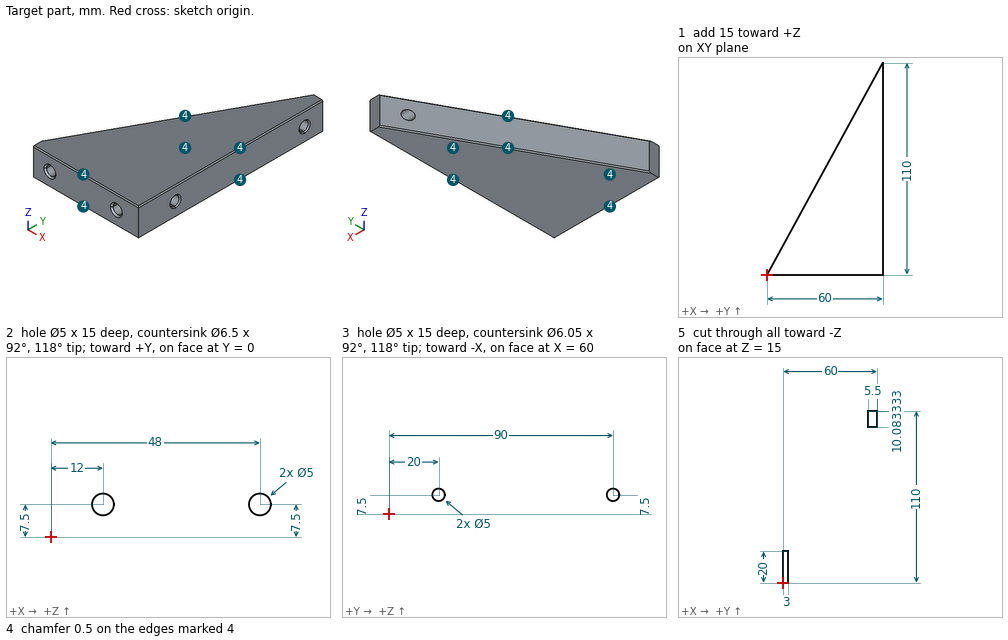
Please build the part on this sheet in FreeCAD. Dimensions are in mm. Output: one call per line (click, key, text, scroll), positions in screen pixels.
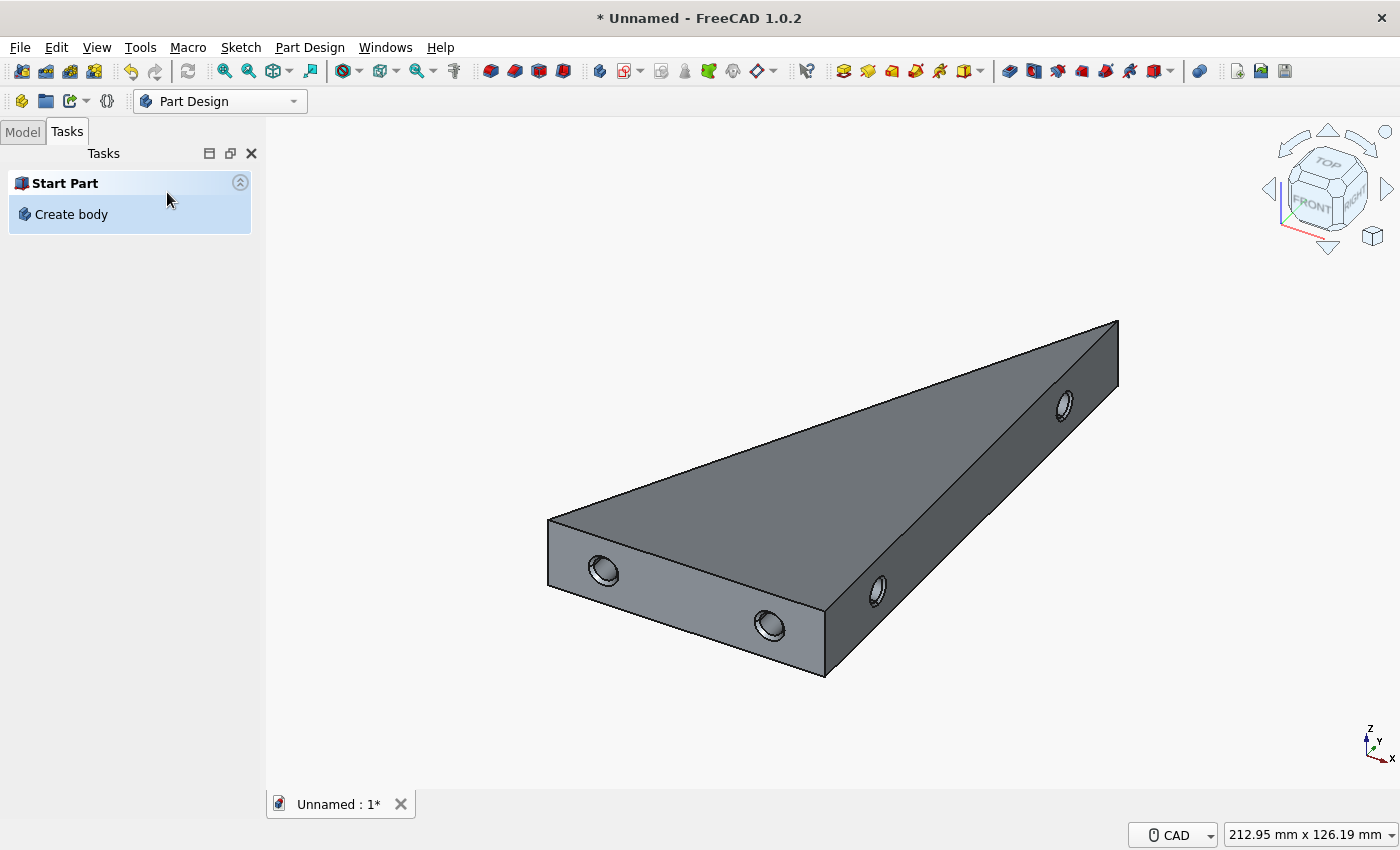
click(789, 516)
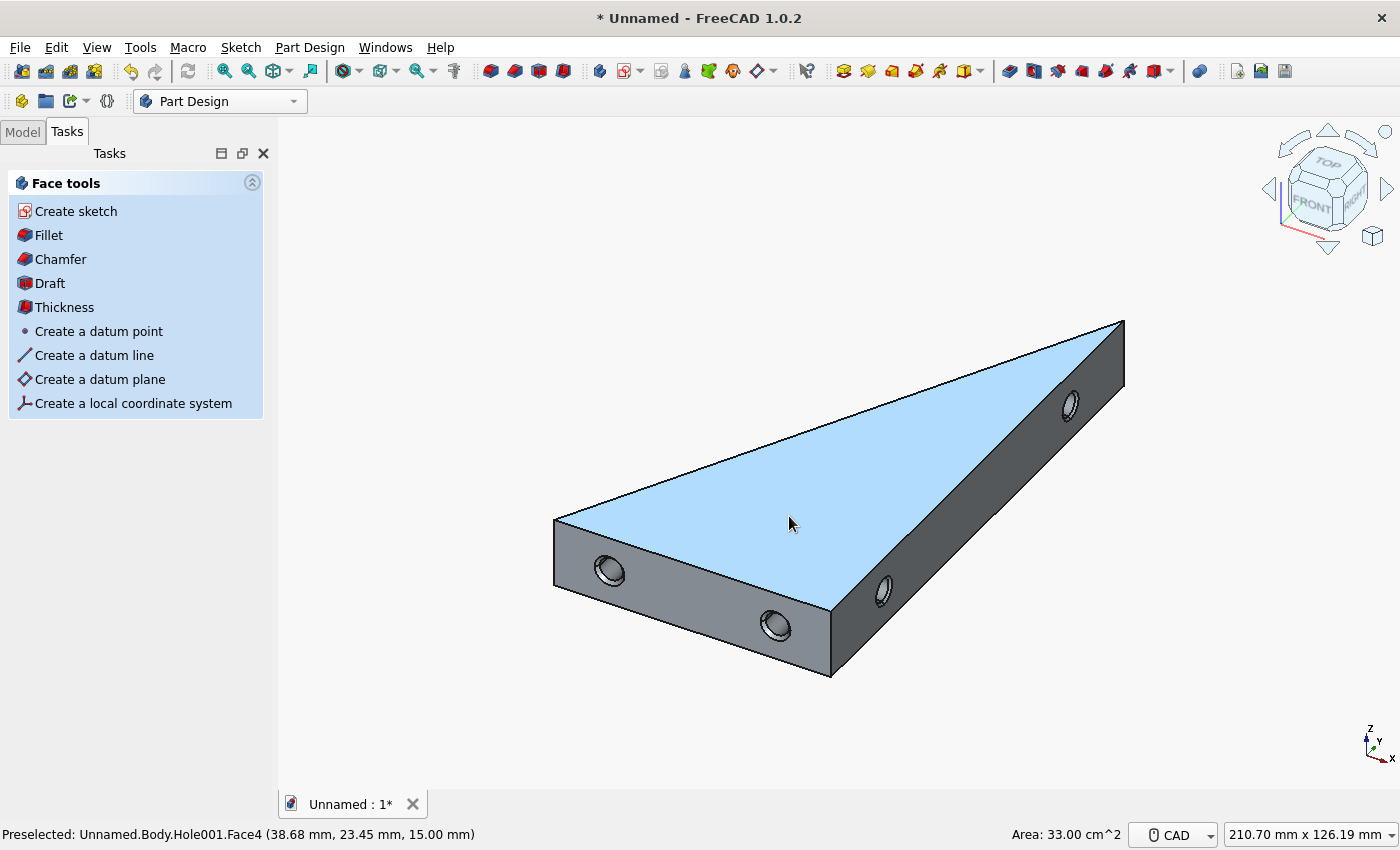
key(0)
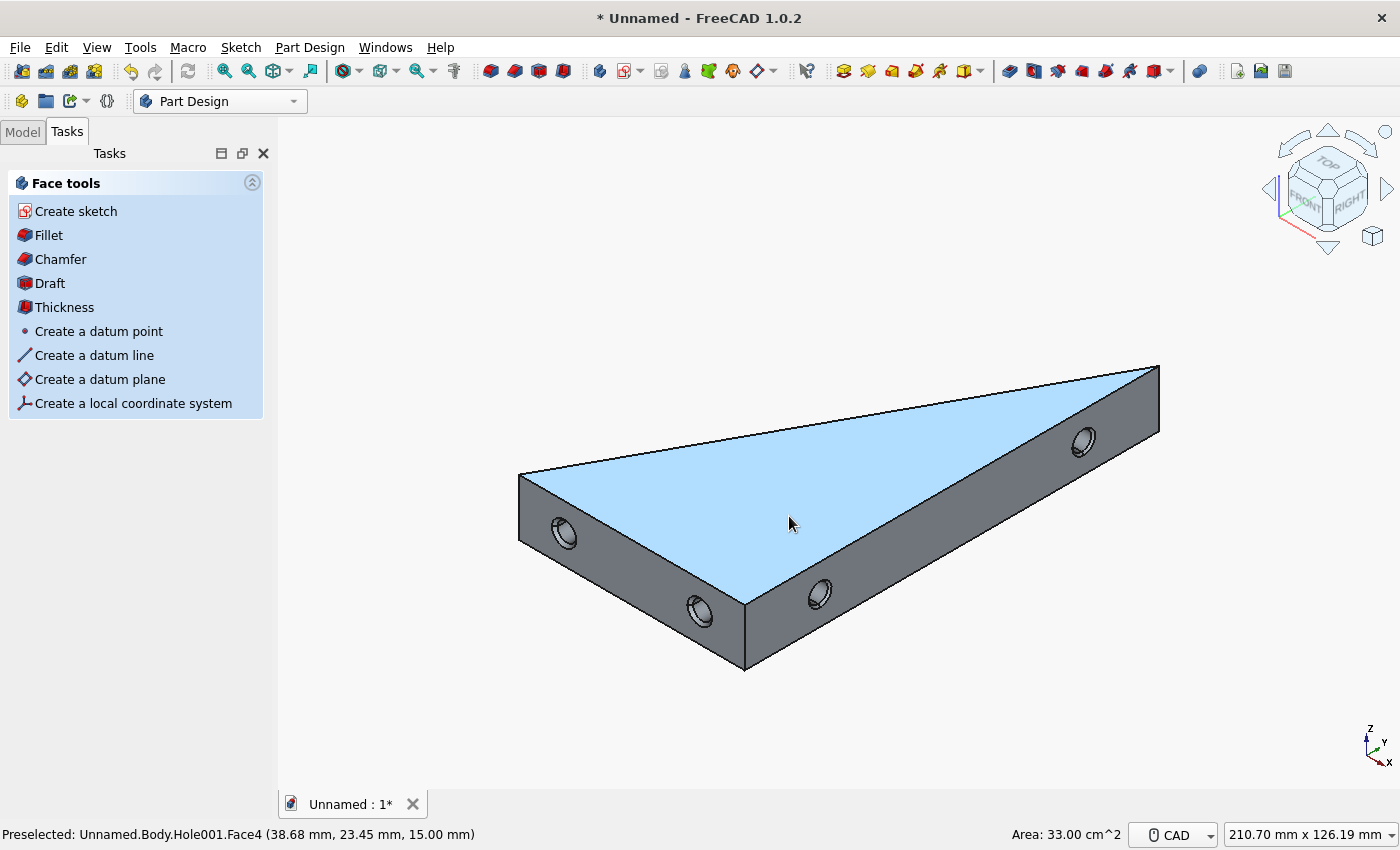
key(2)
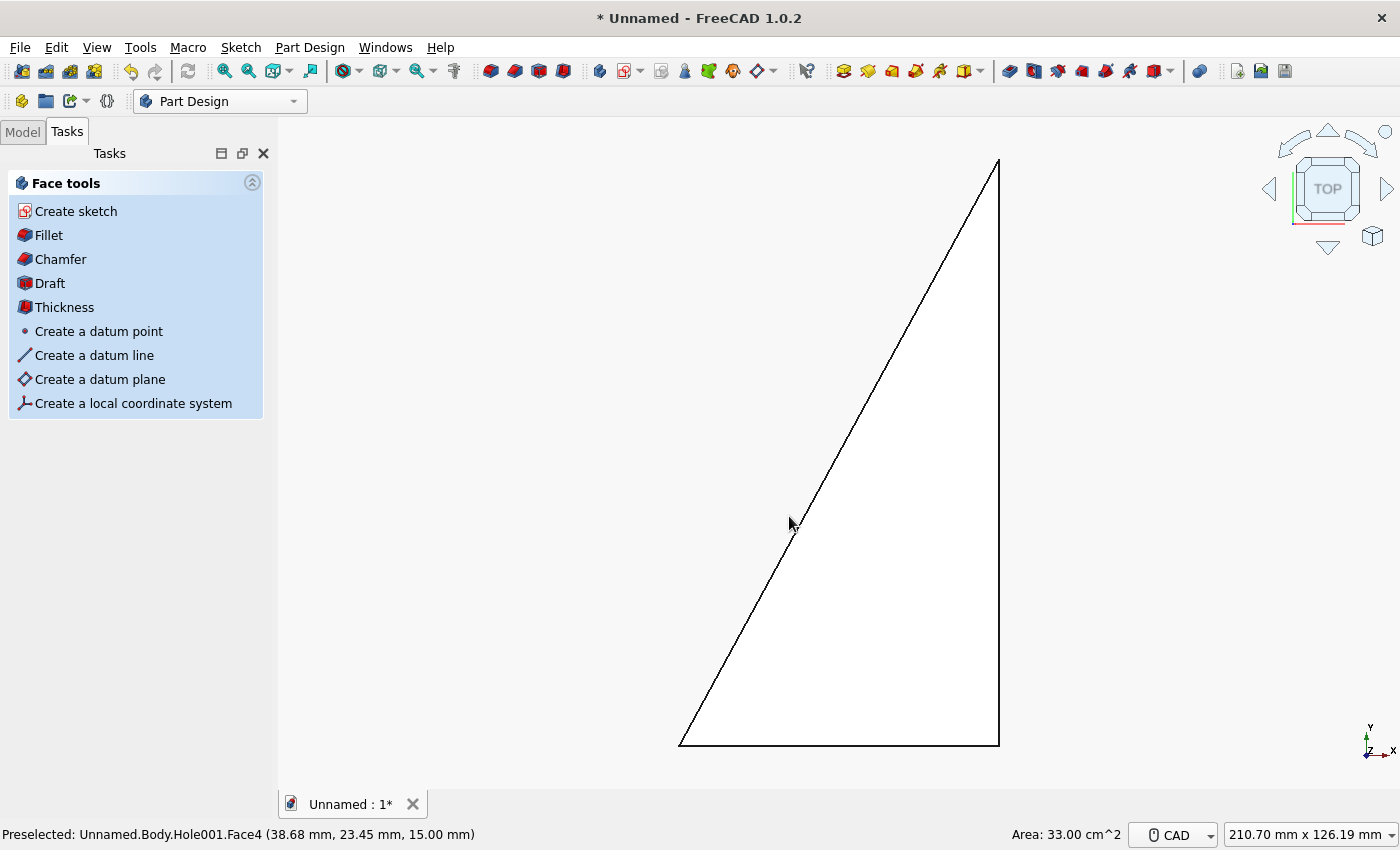
key(1)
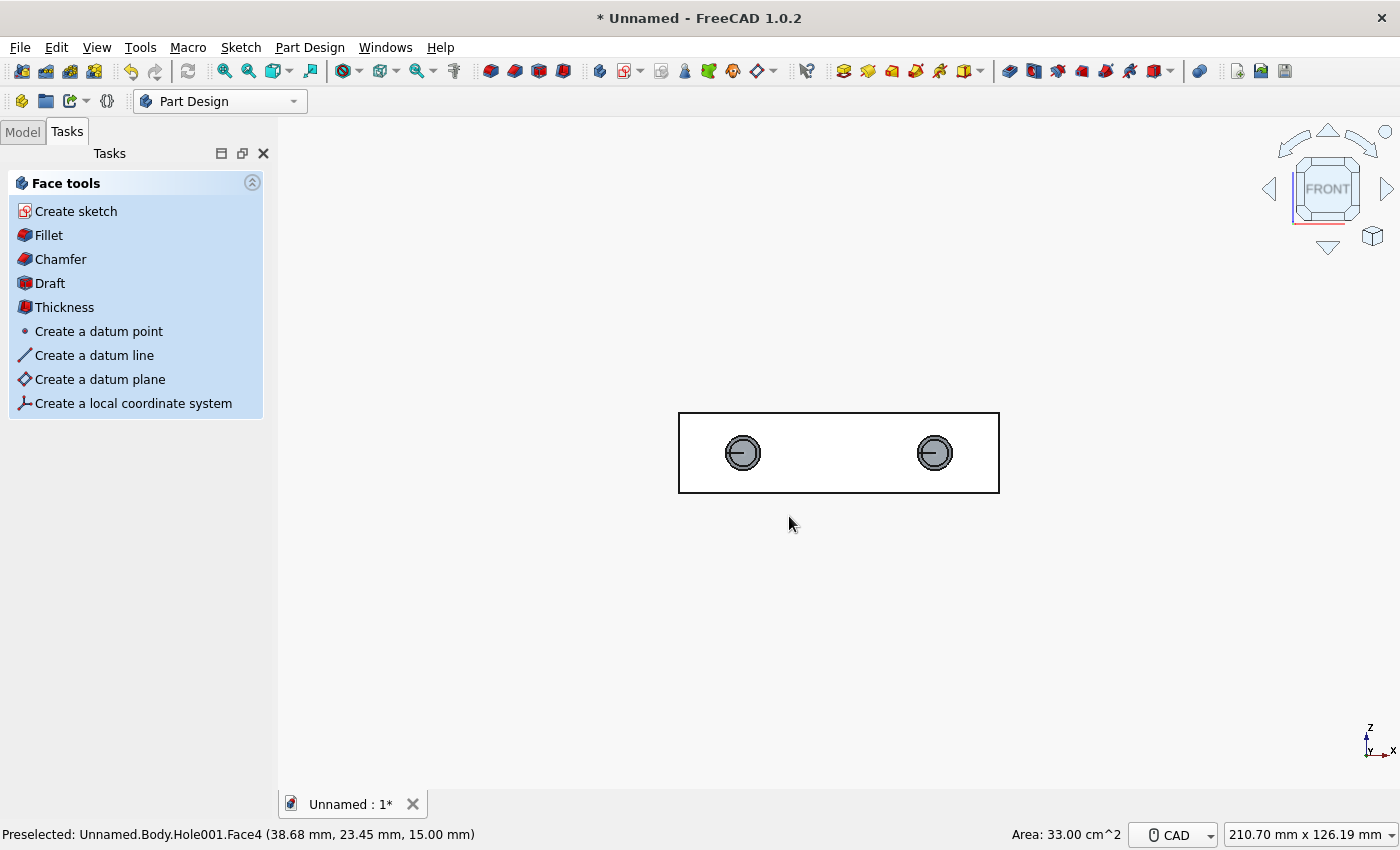
click(226, 72)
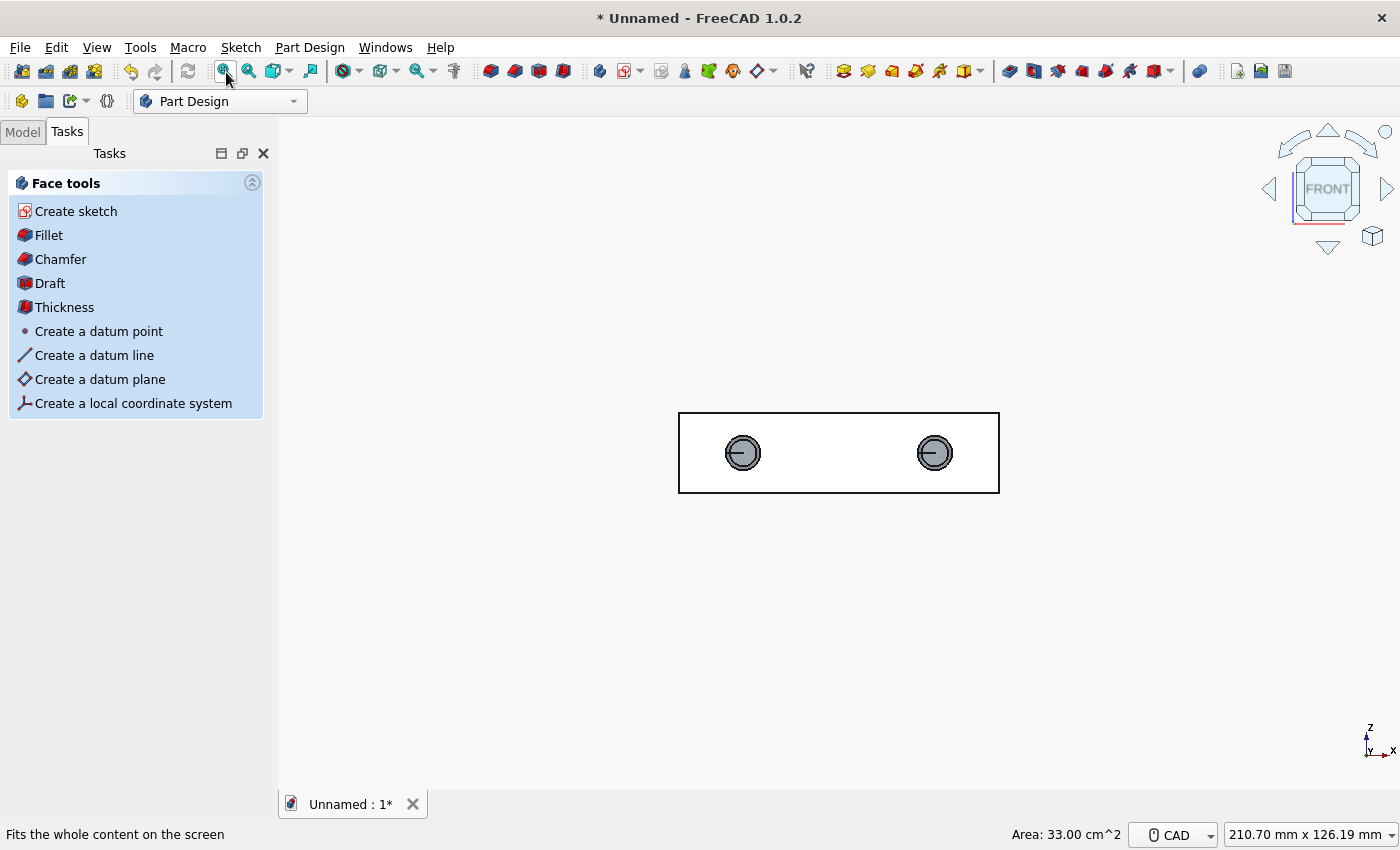
key(3)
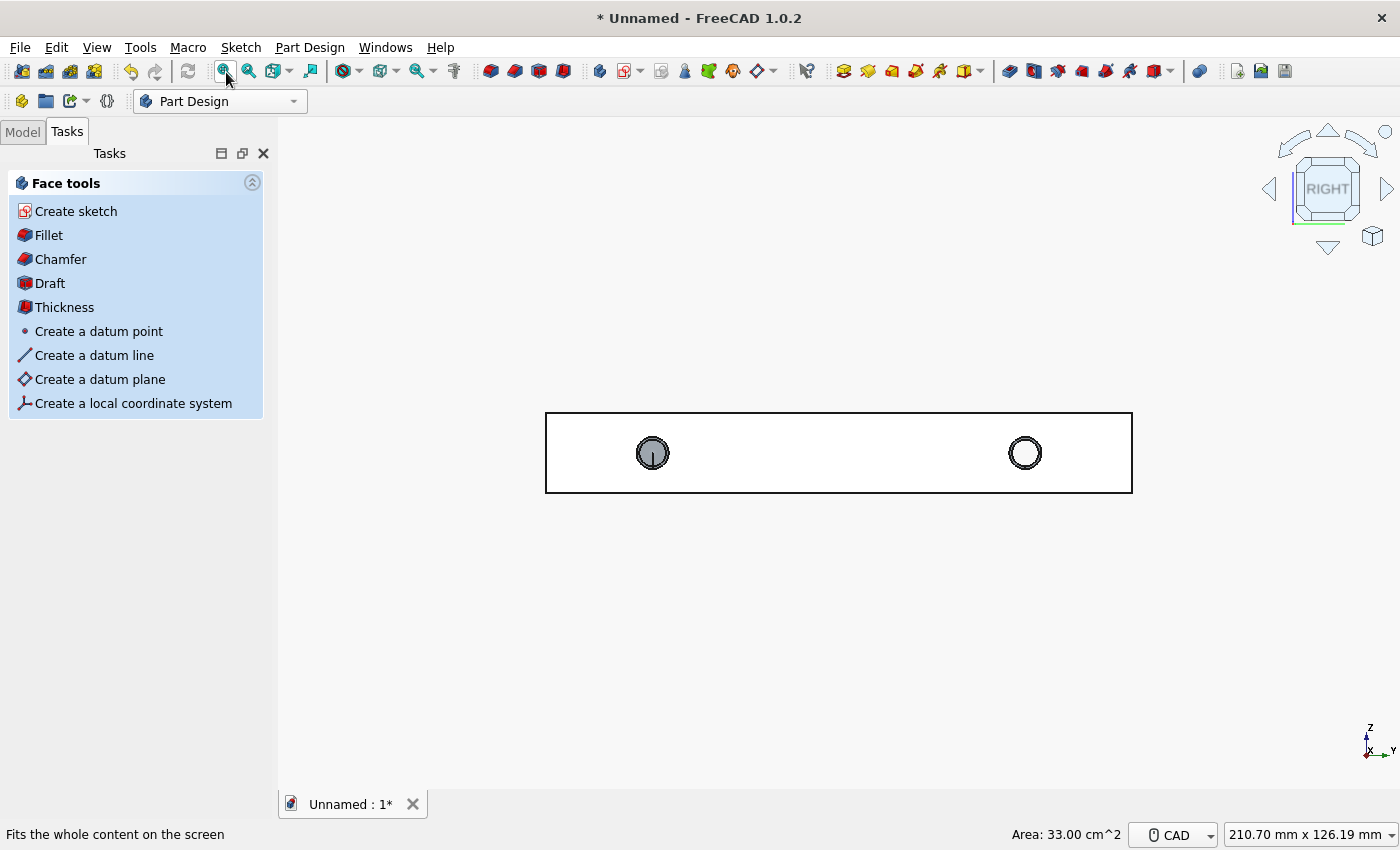
key(5)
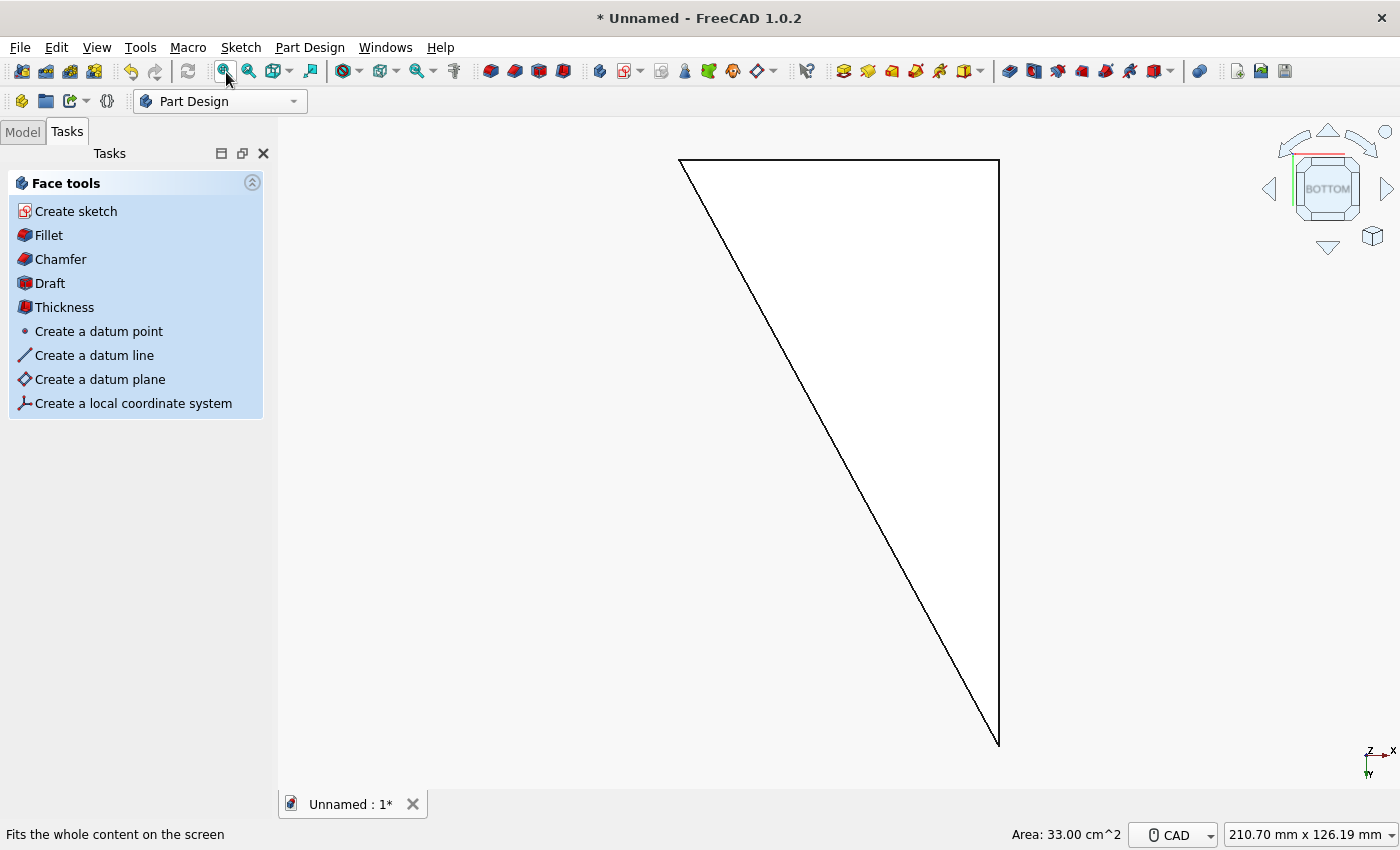
click(885, 285, ctrl)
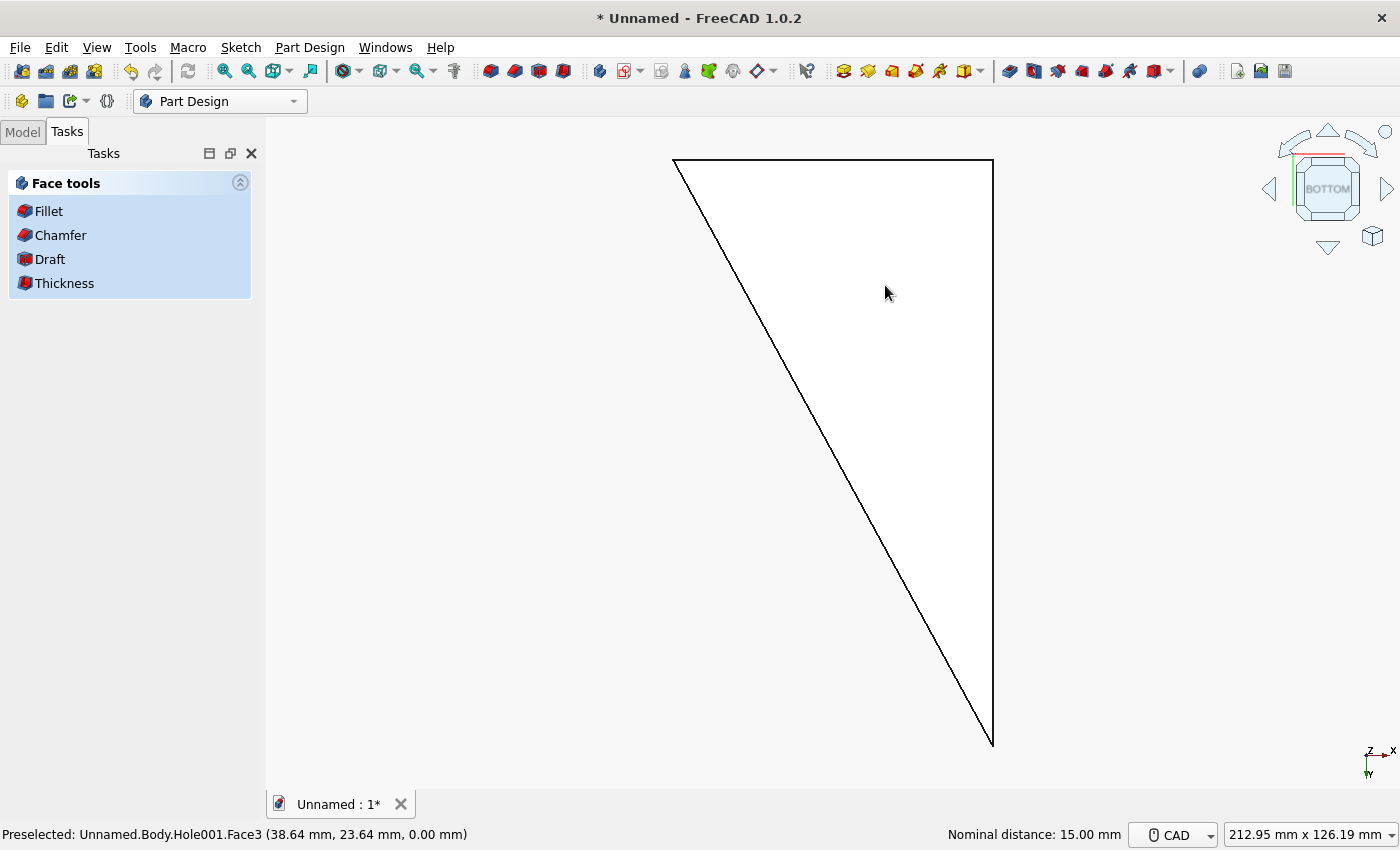
click(516, 72)